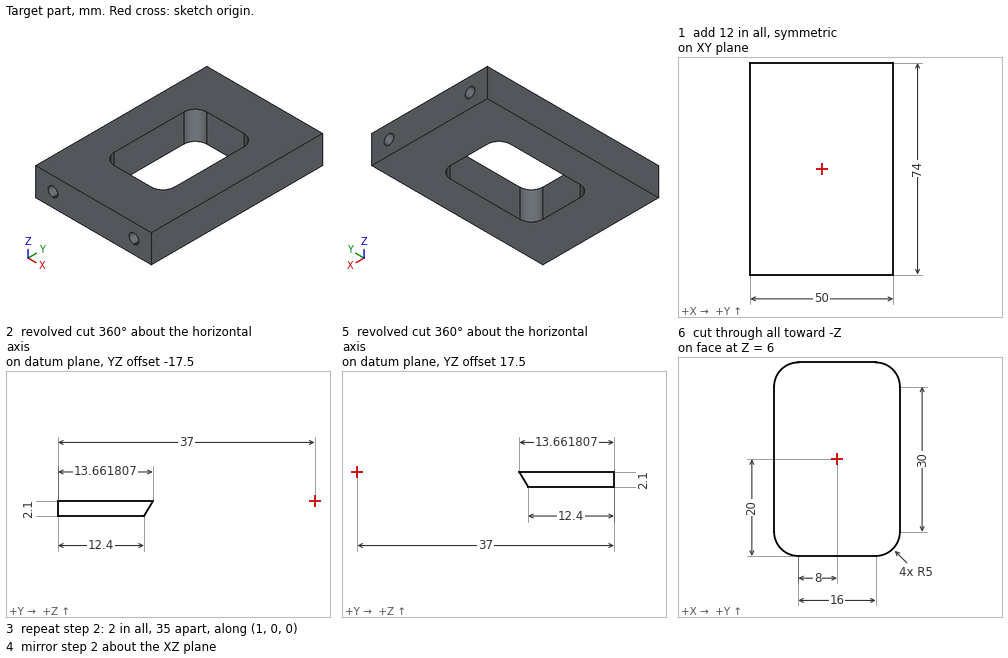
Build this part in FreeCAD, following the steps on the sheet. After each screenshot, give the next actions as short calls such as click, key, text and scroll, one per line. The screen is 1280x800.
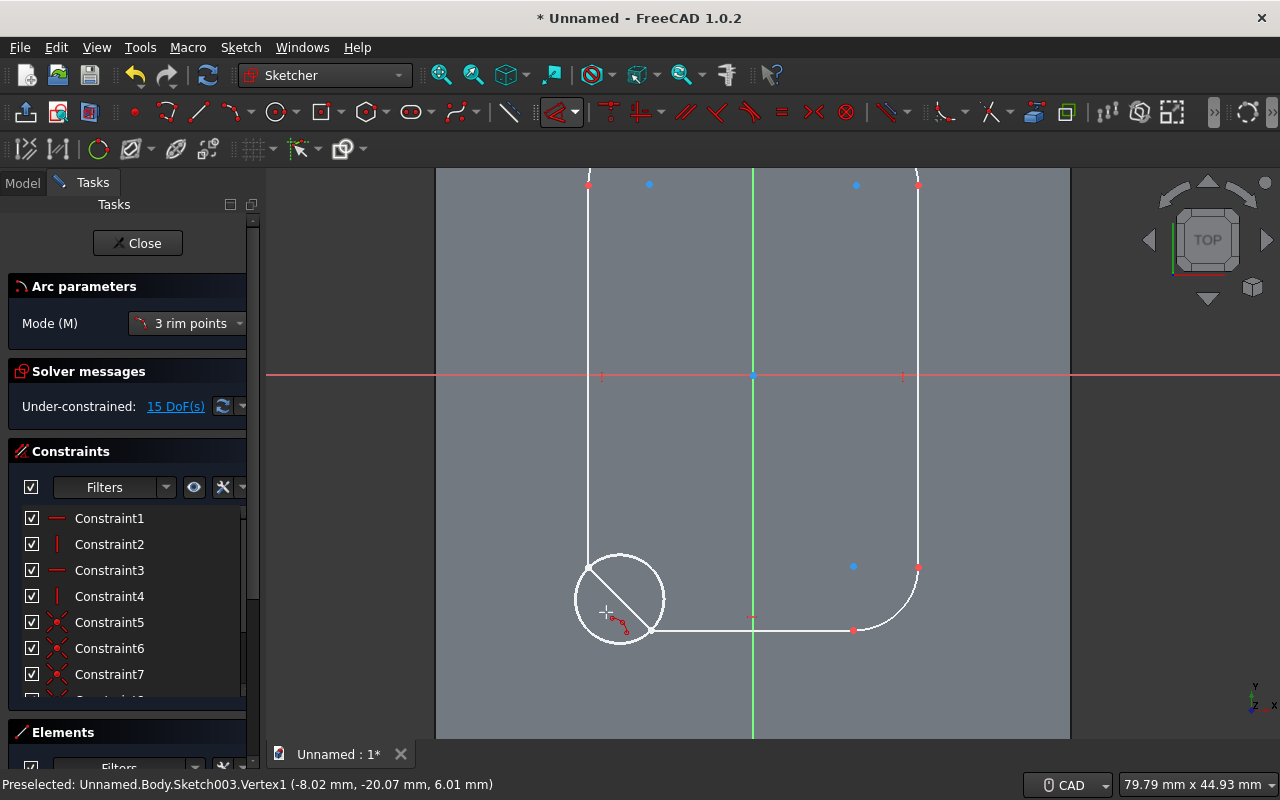
click(606, 611)
key(Escape)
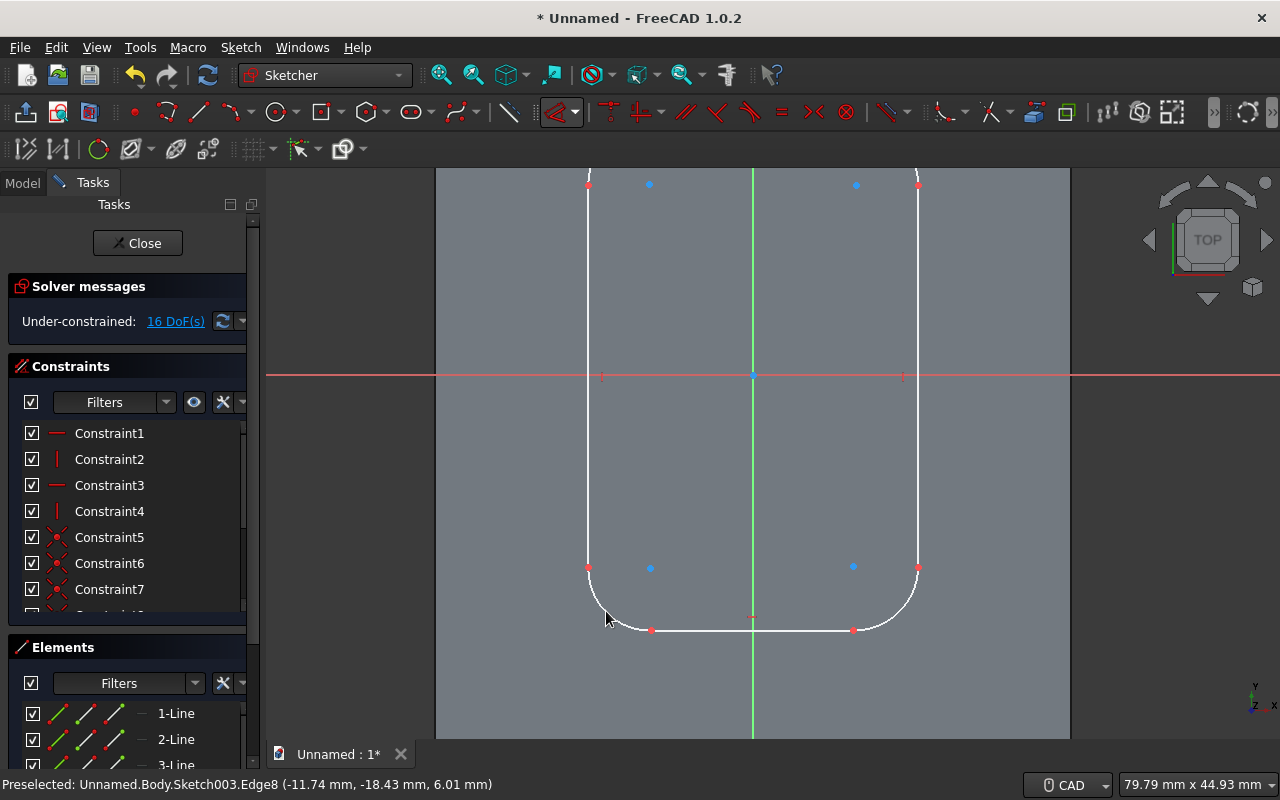
click(712, 631)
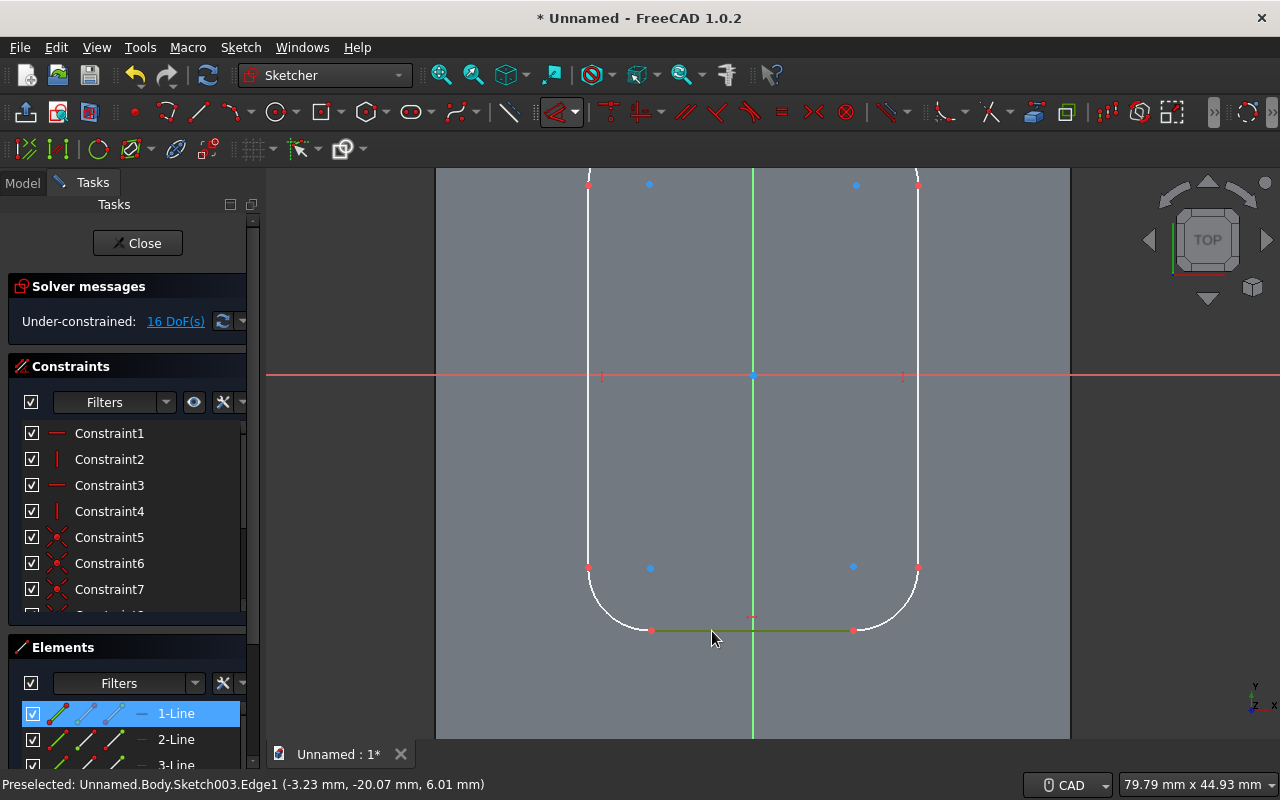
click(883, 624)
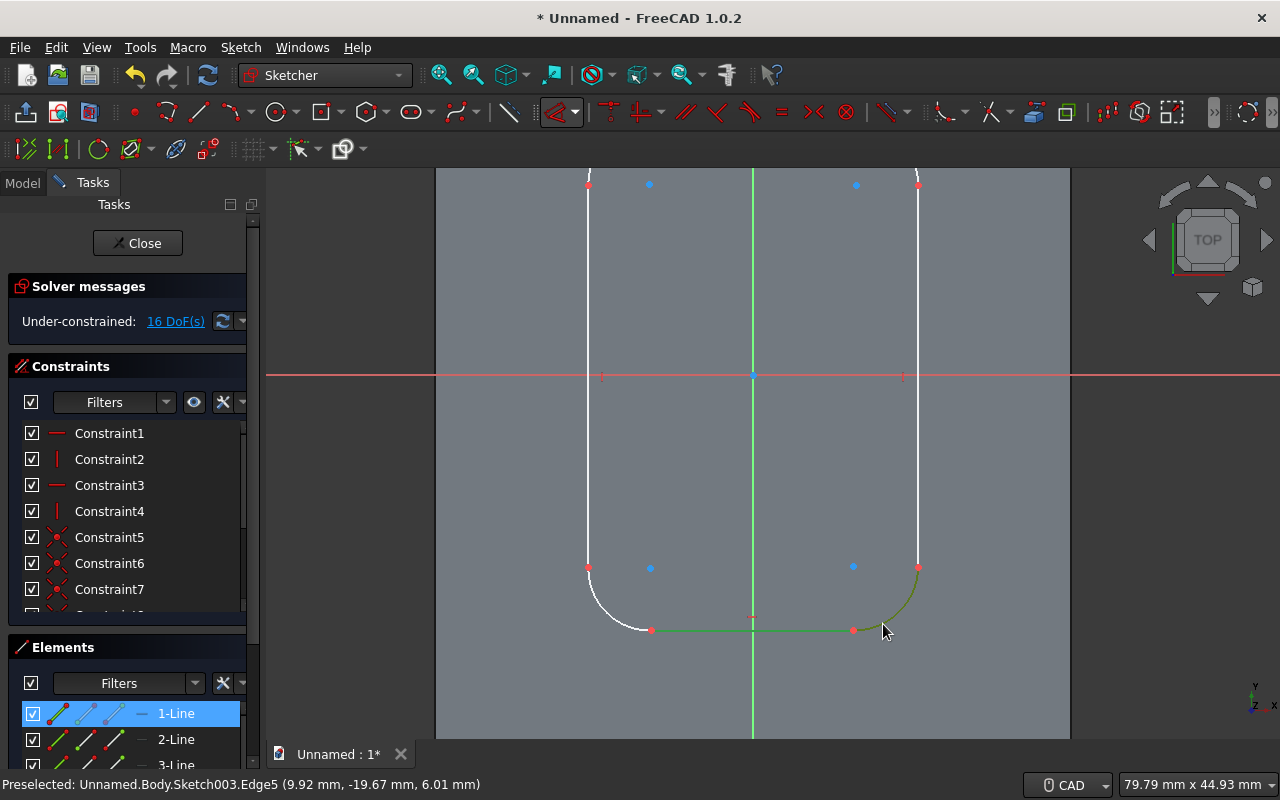
click(750, 112)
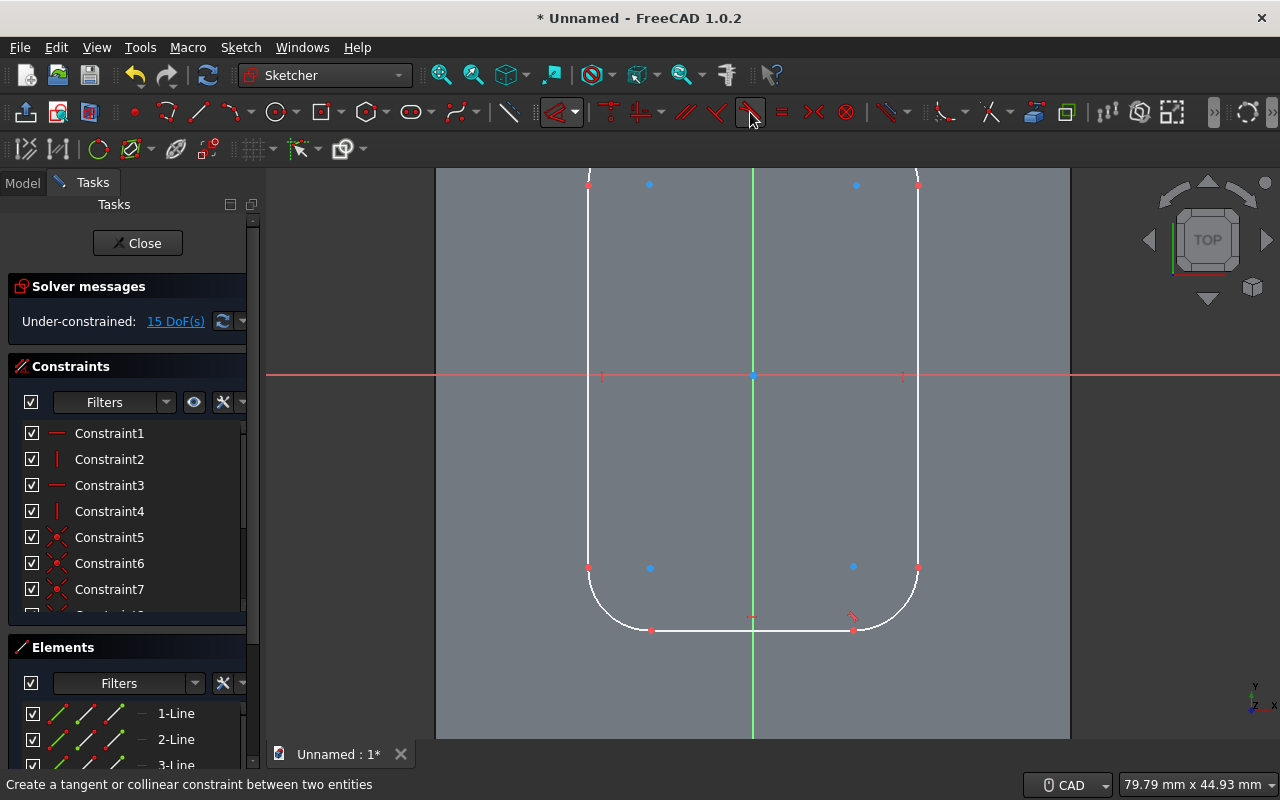
click(712, 631)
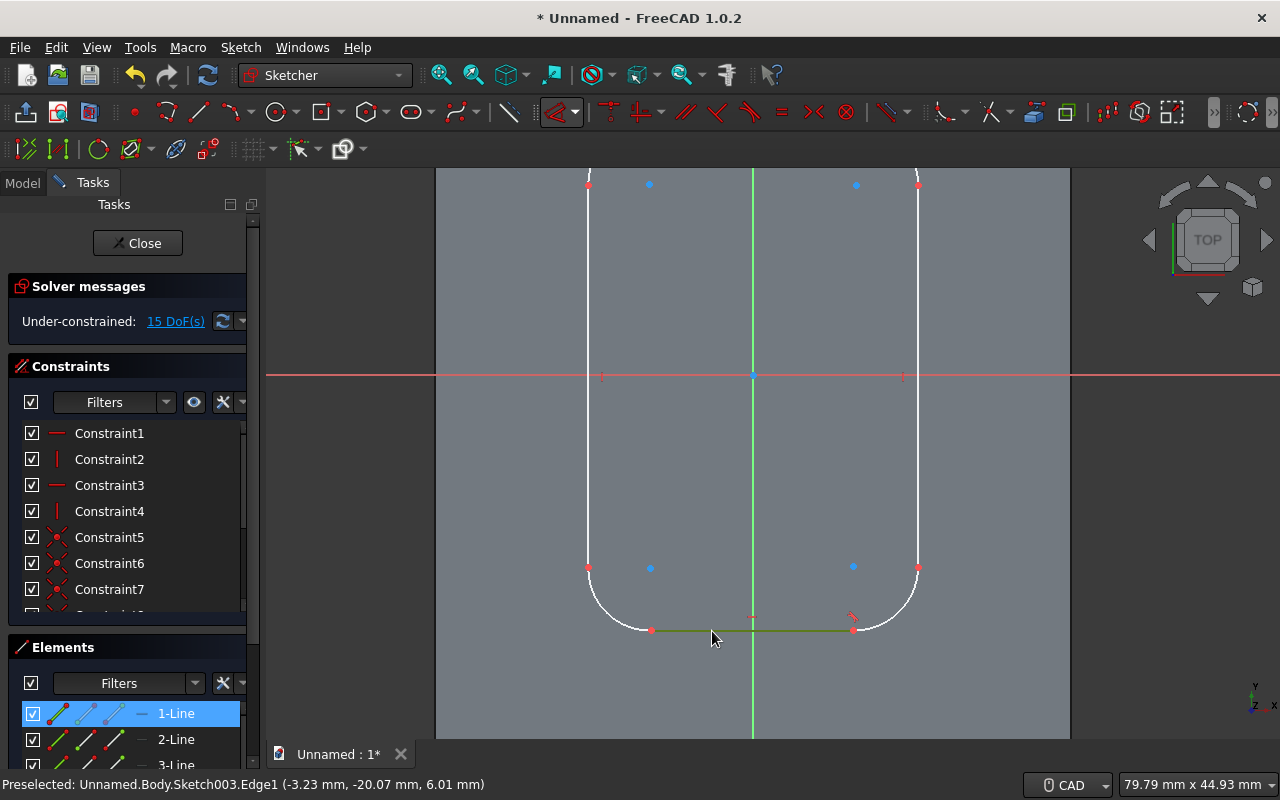
click(595, 596)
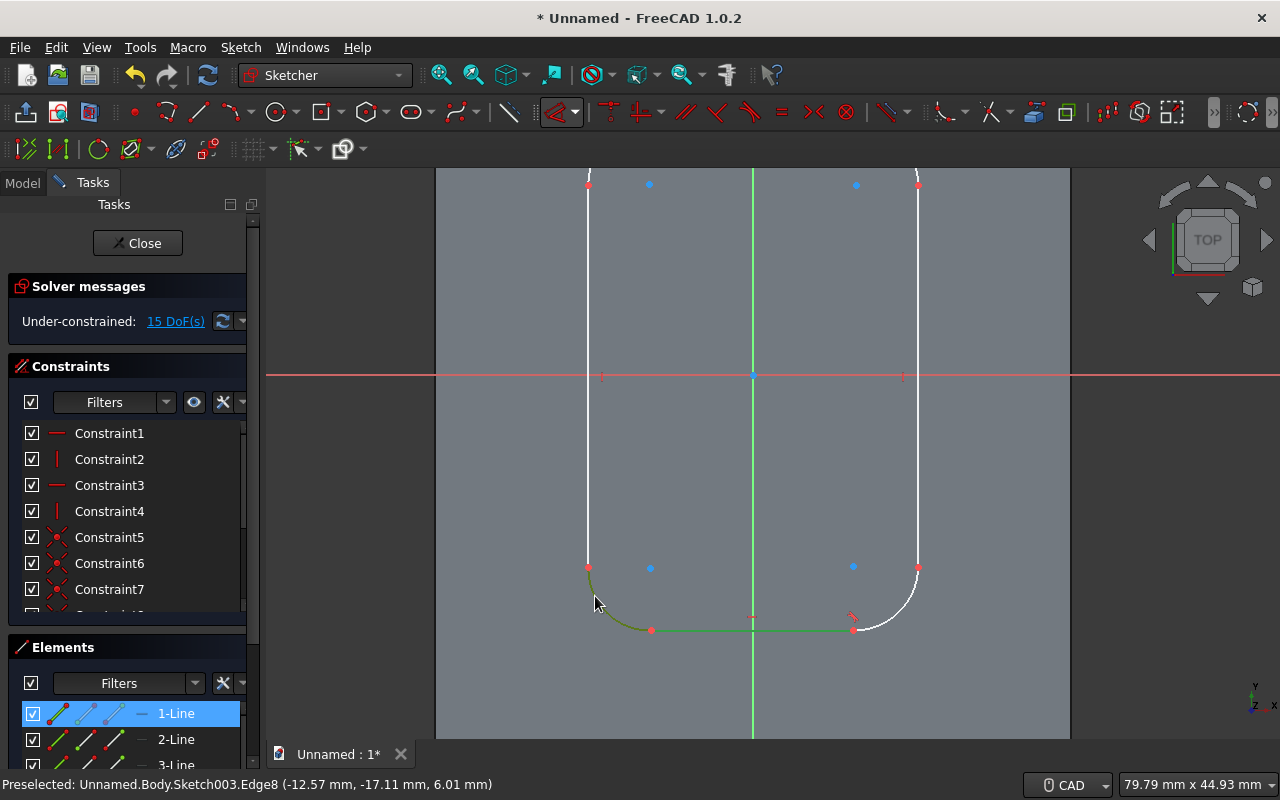
key(t)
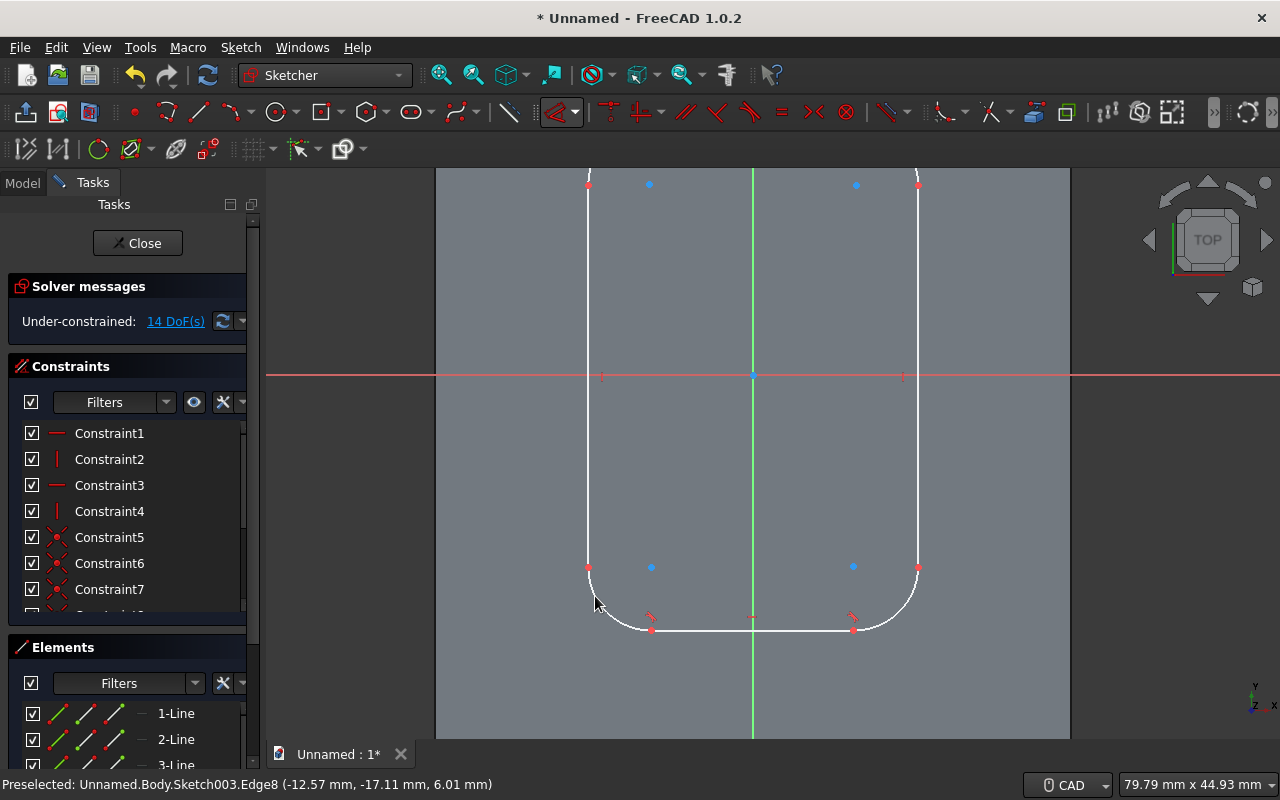
click(918, 453)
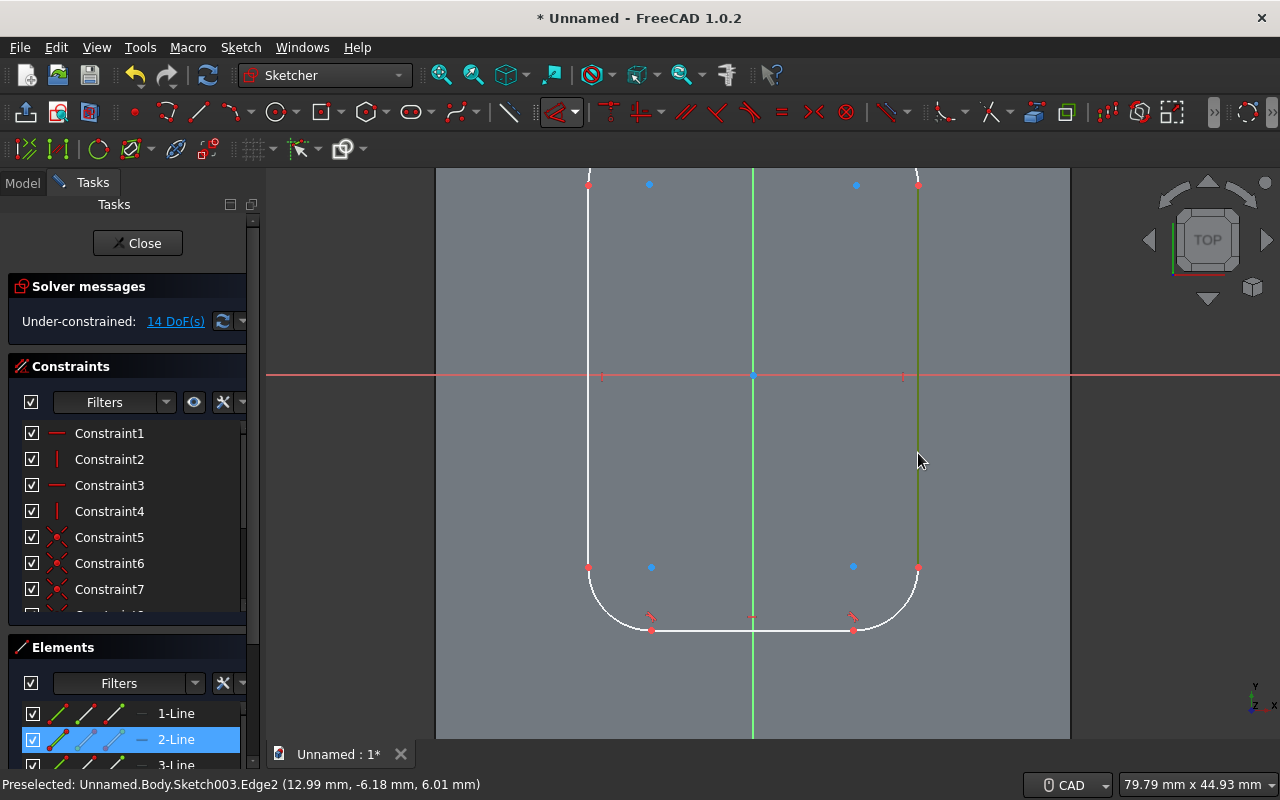
click(883, 624)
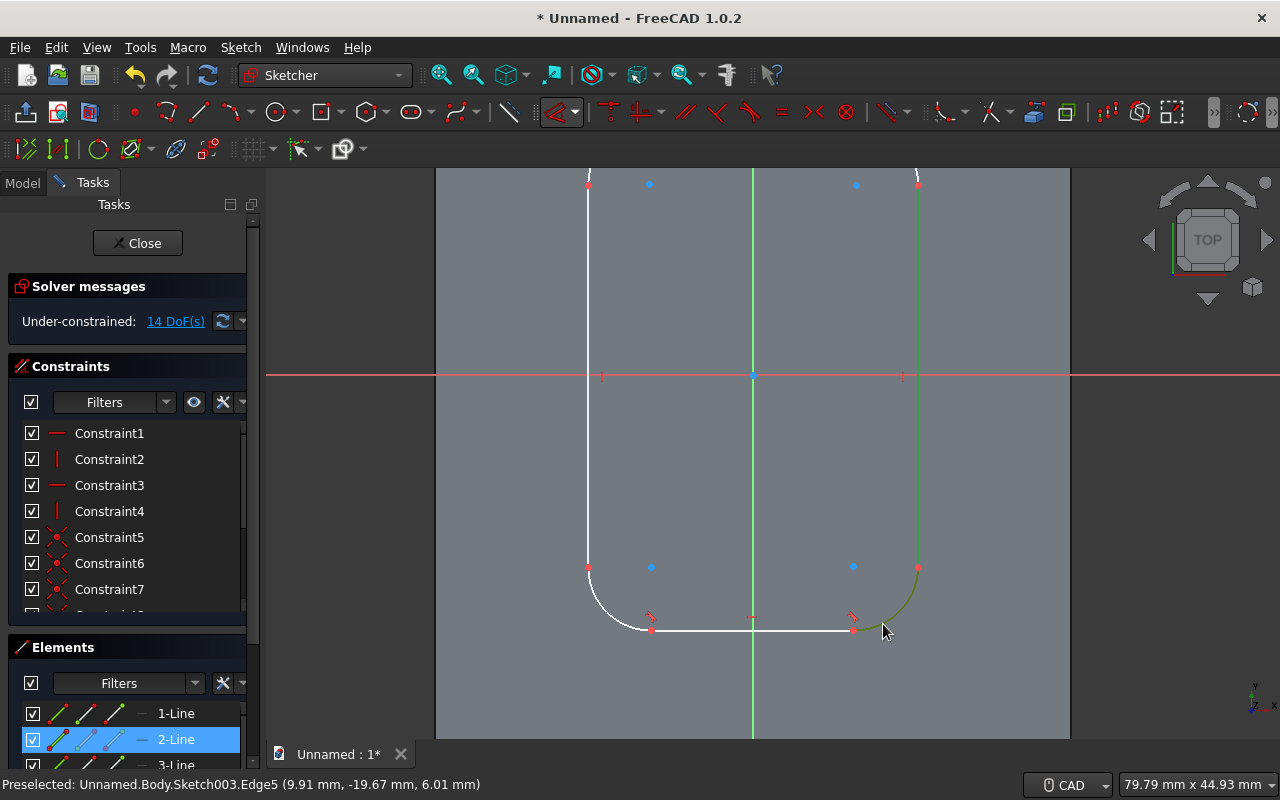
click(750, 112)